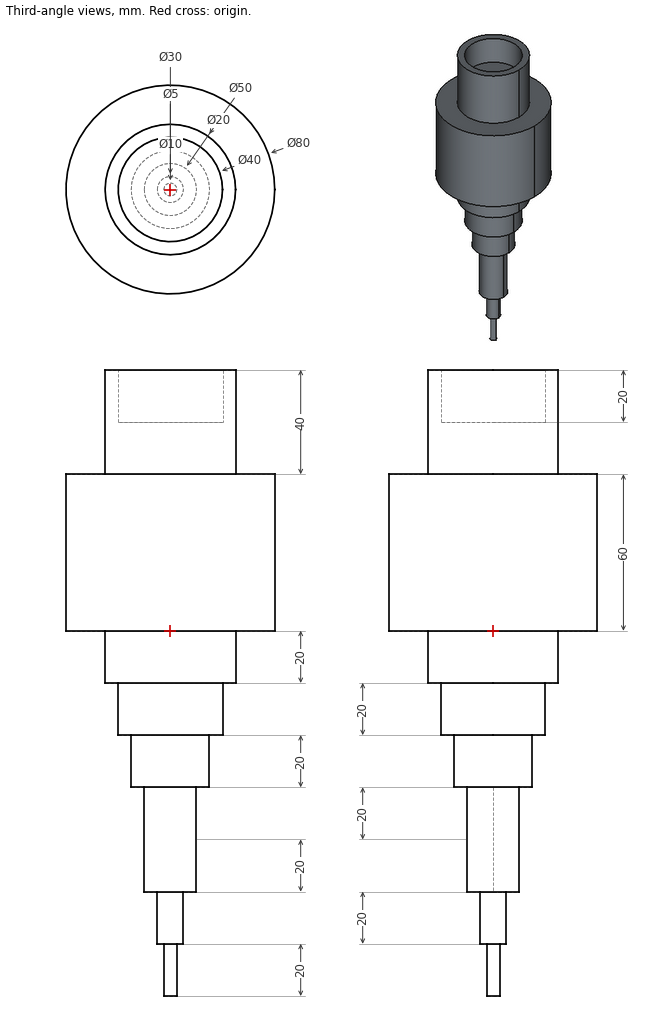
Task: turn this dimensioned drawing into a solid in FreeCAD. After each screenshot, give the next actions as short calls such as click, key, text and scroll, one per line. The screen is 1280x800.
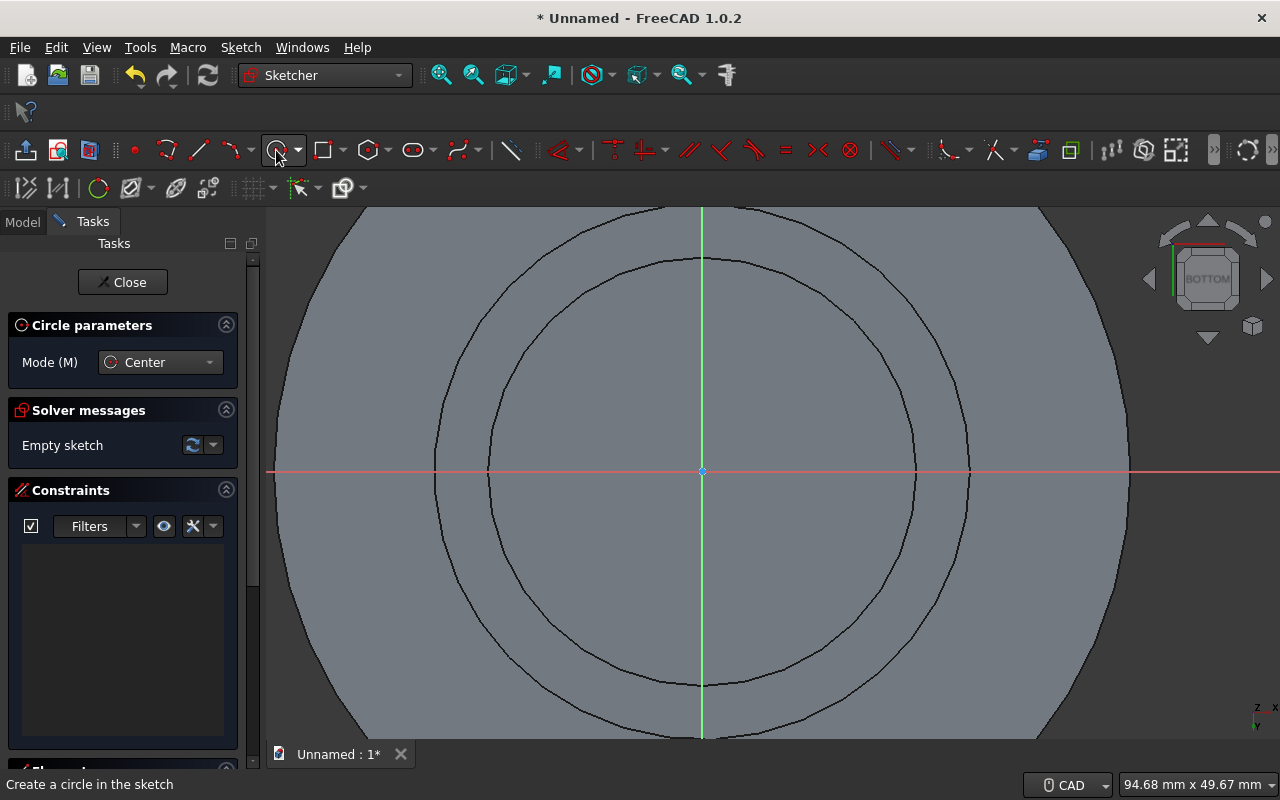
click(702, 472)
click(816, 358)
key(Escape)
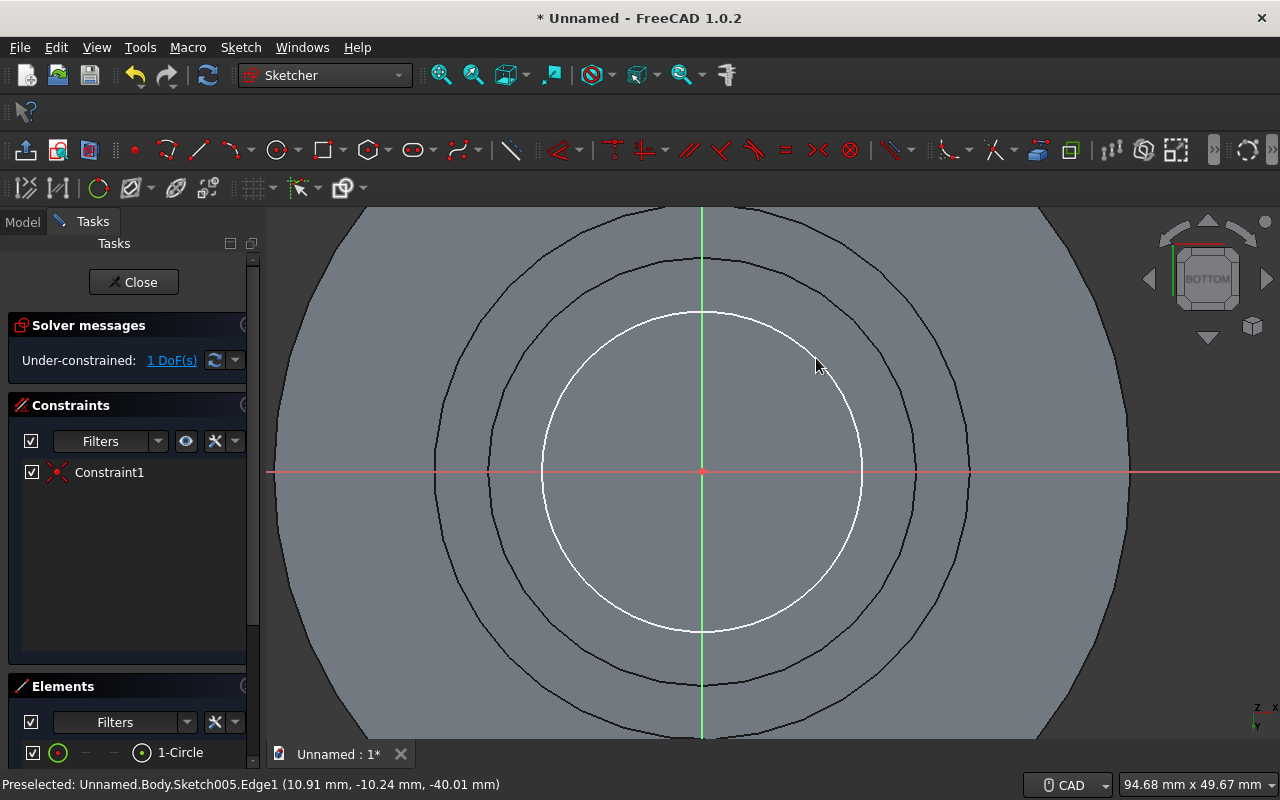
key(d)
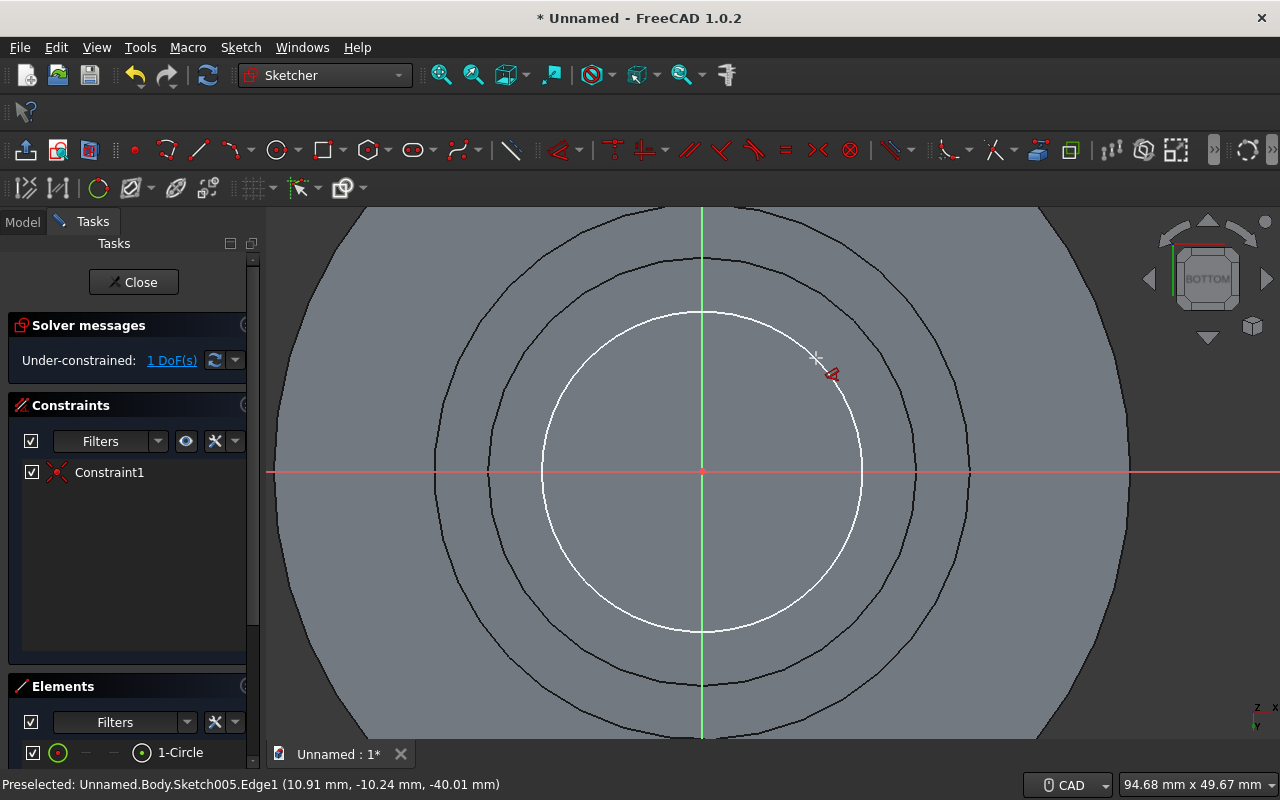
click(815, 358)
click(838, 335)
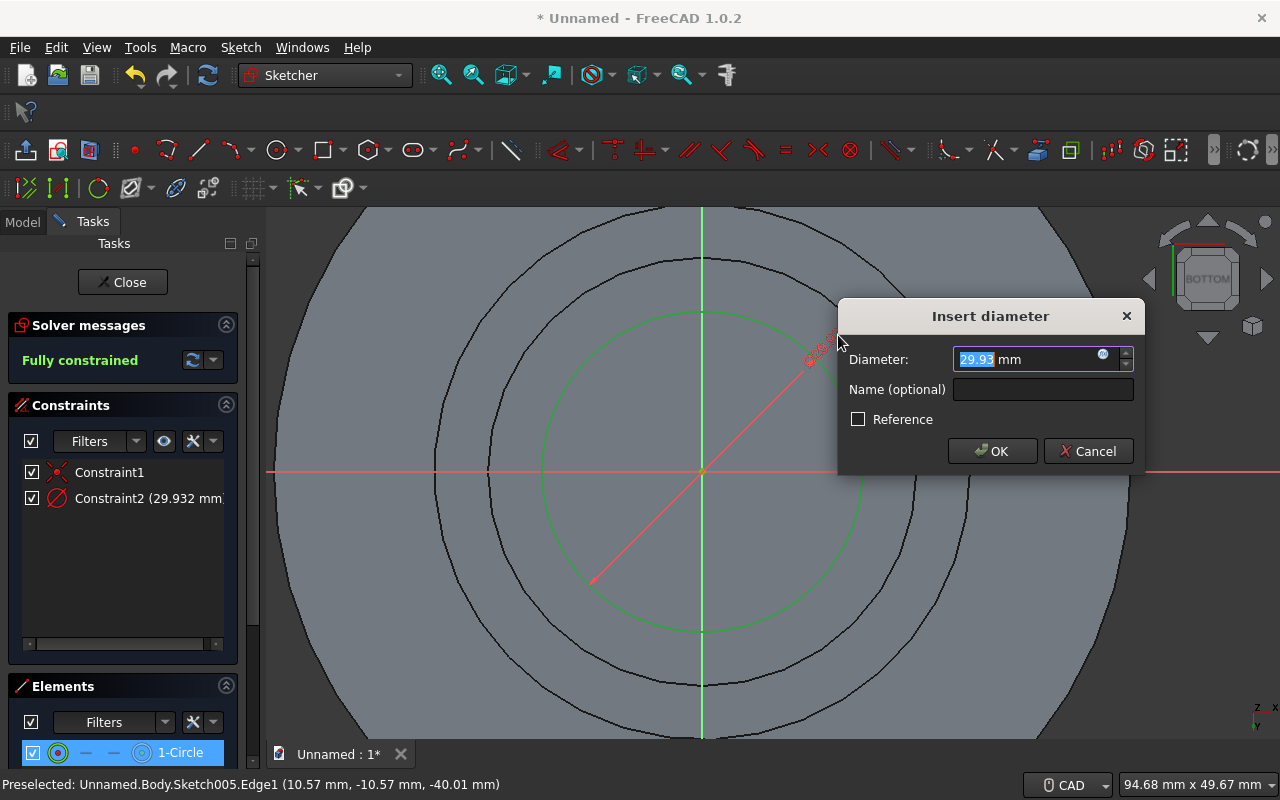
text(30)
key(Return)
key(Escape)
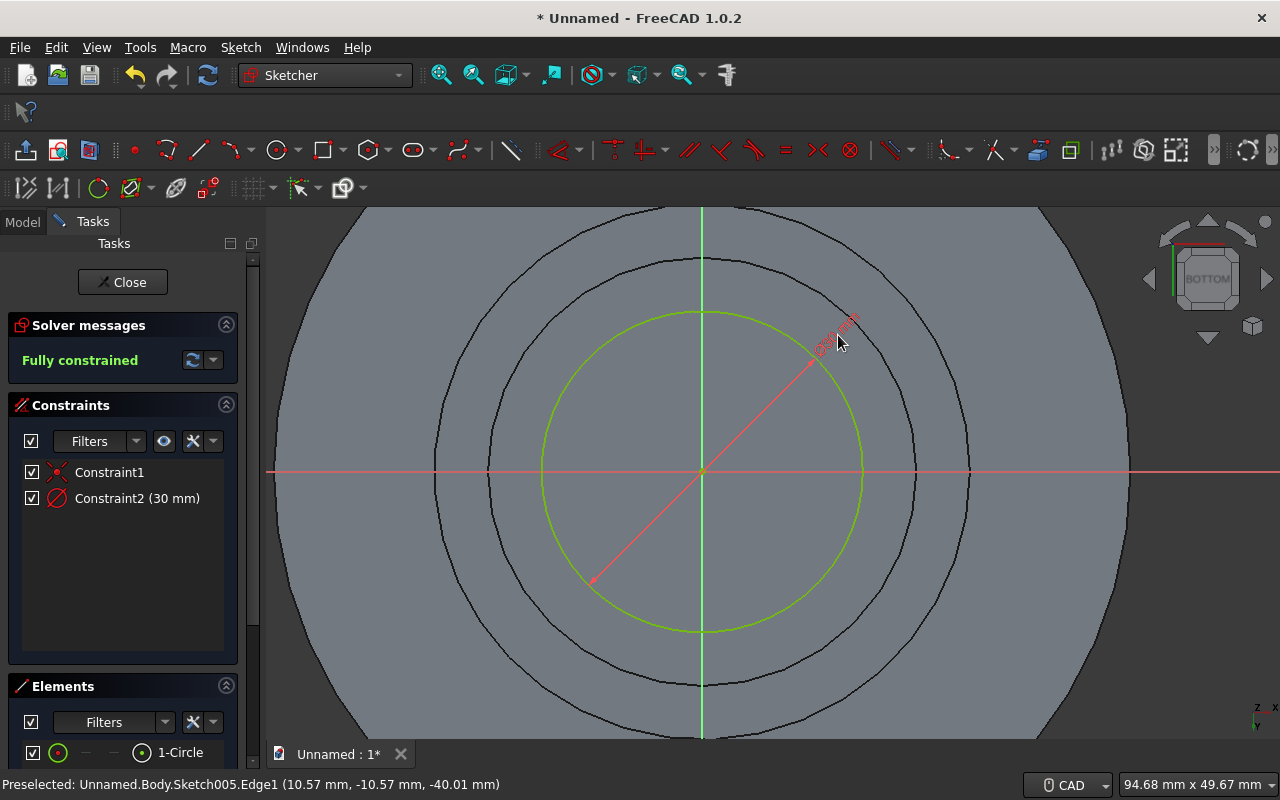
click(123, 282)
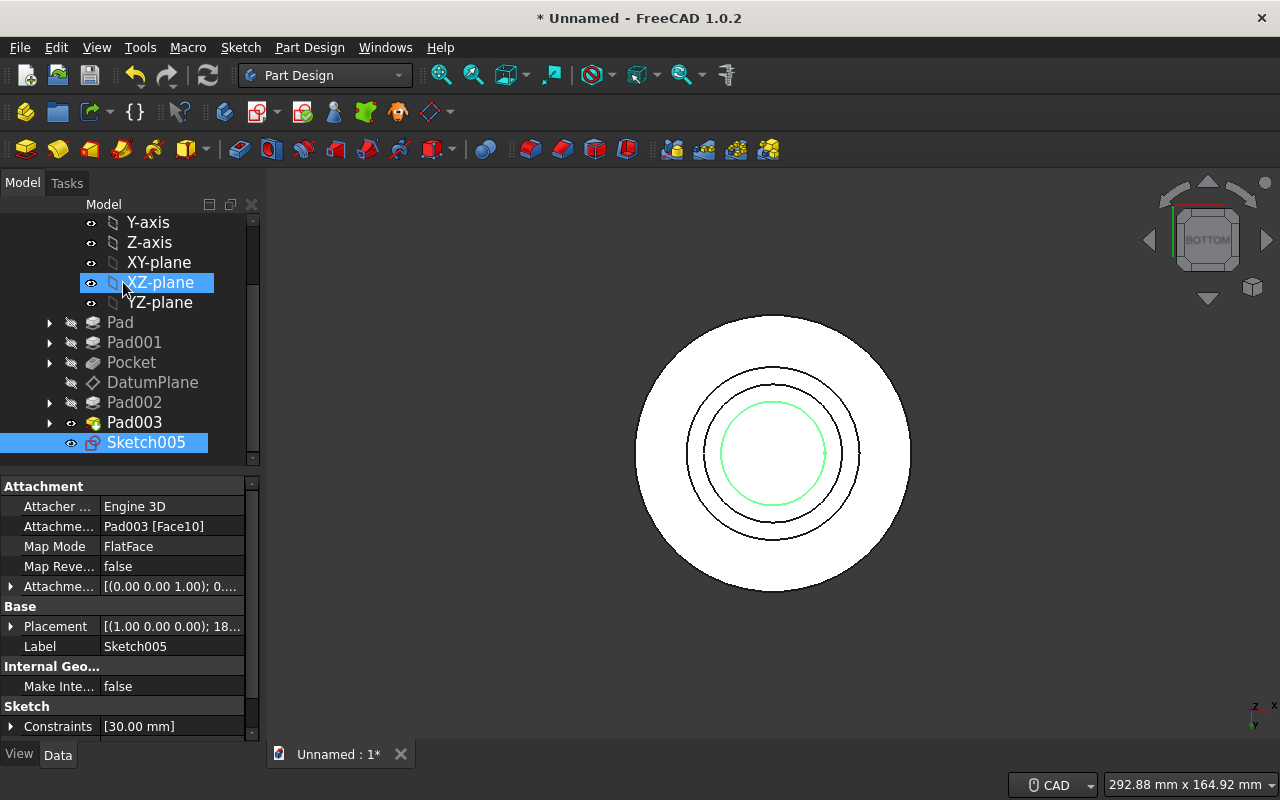
click(26, 150)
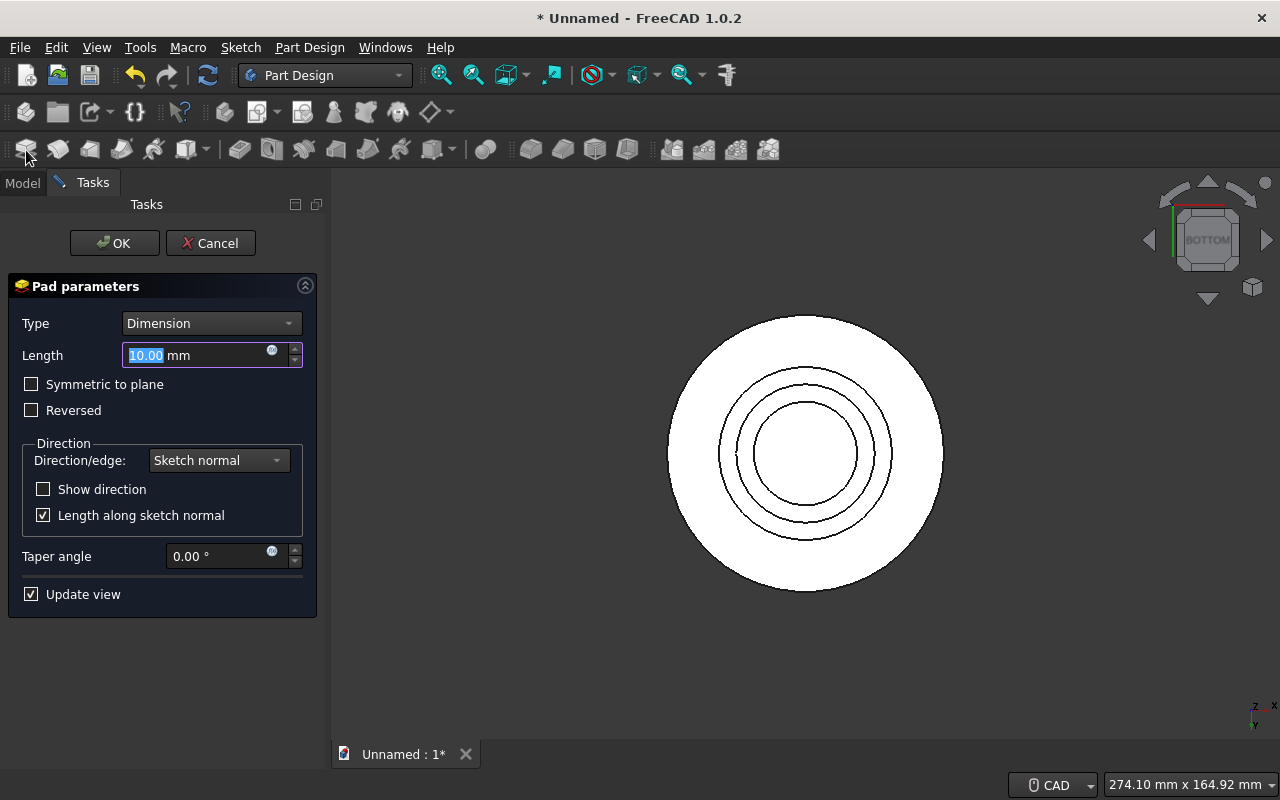
text(20)
key(Tab)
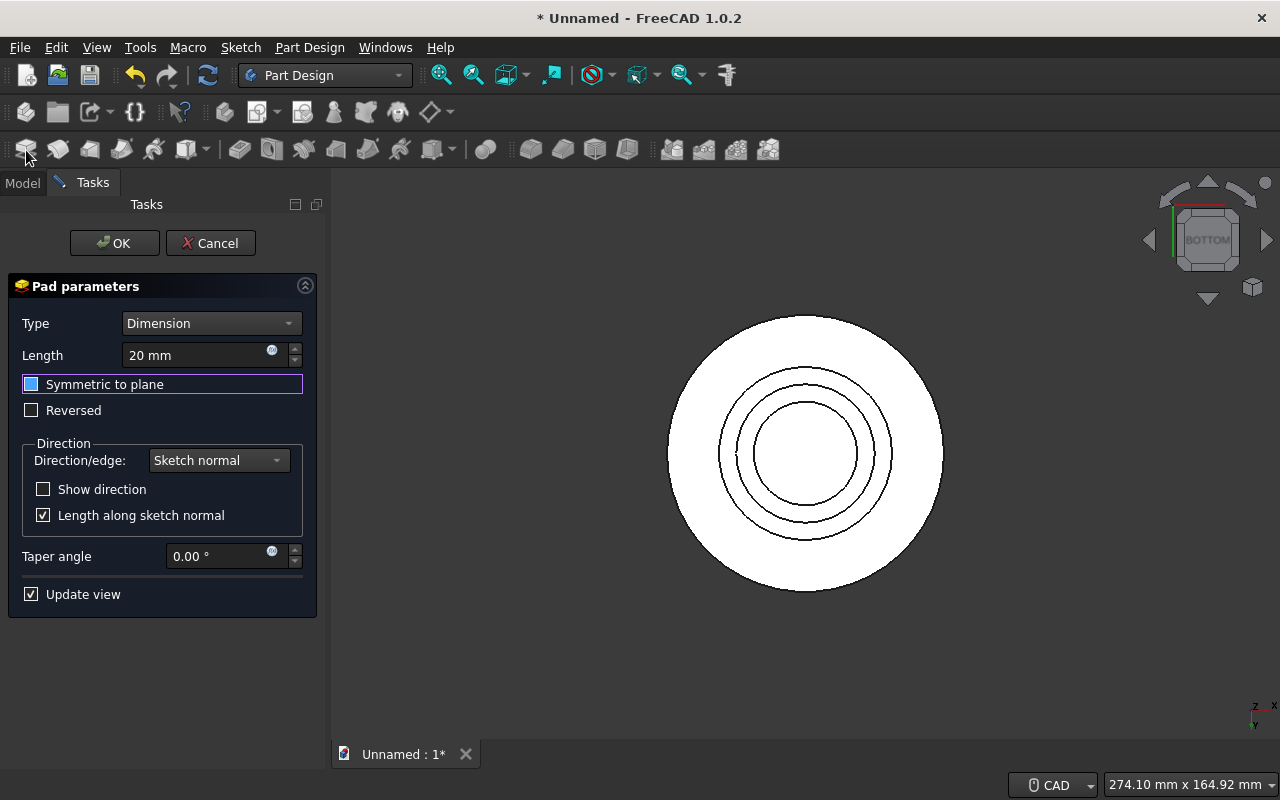
click(115, 243)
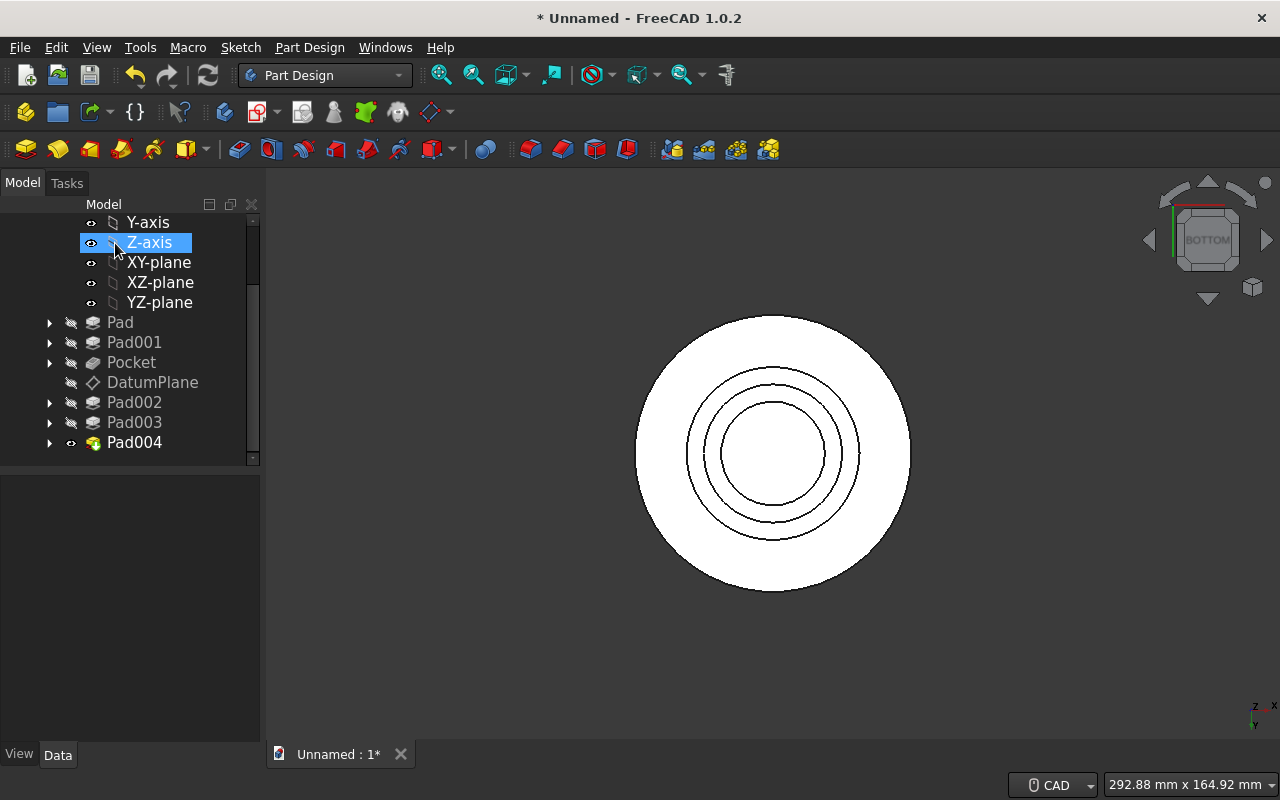
click(773, 452)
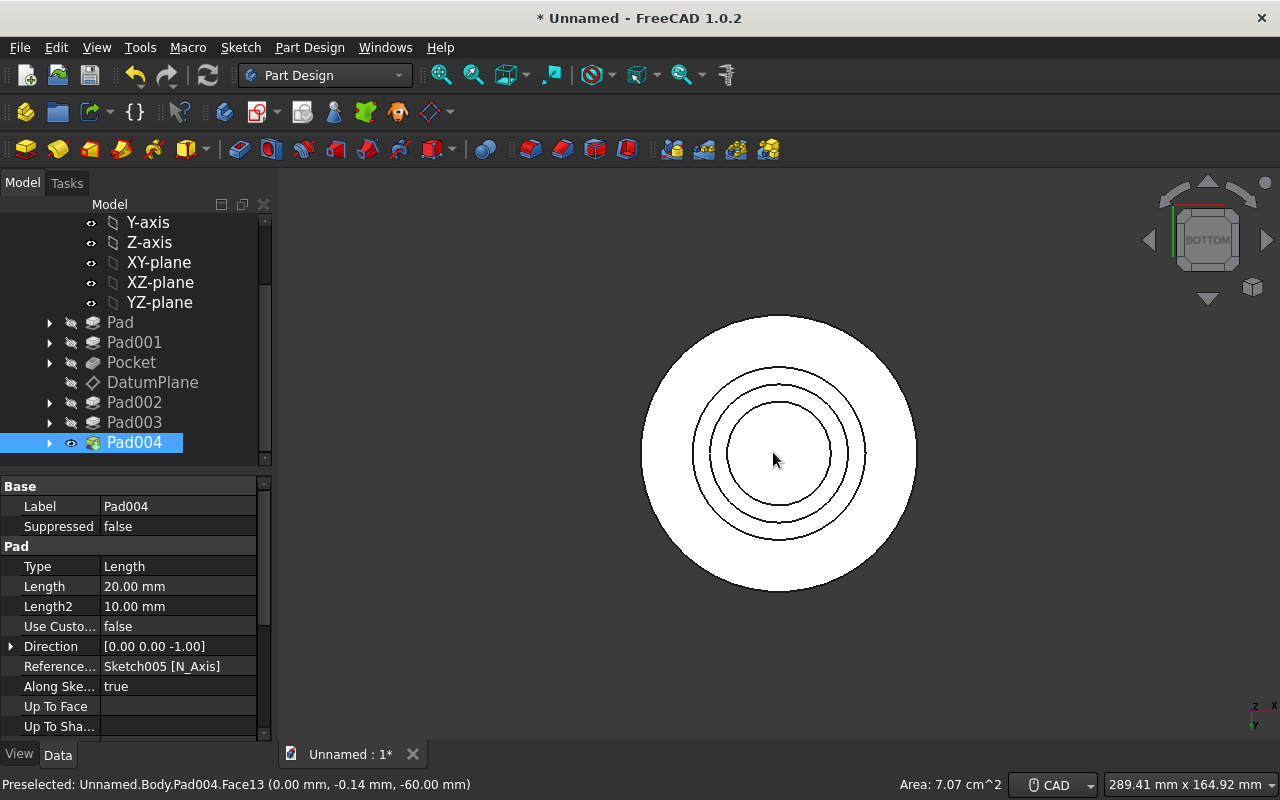
click(258, 112)